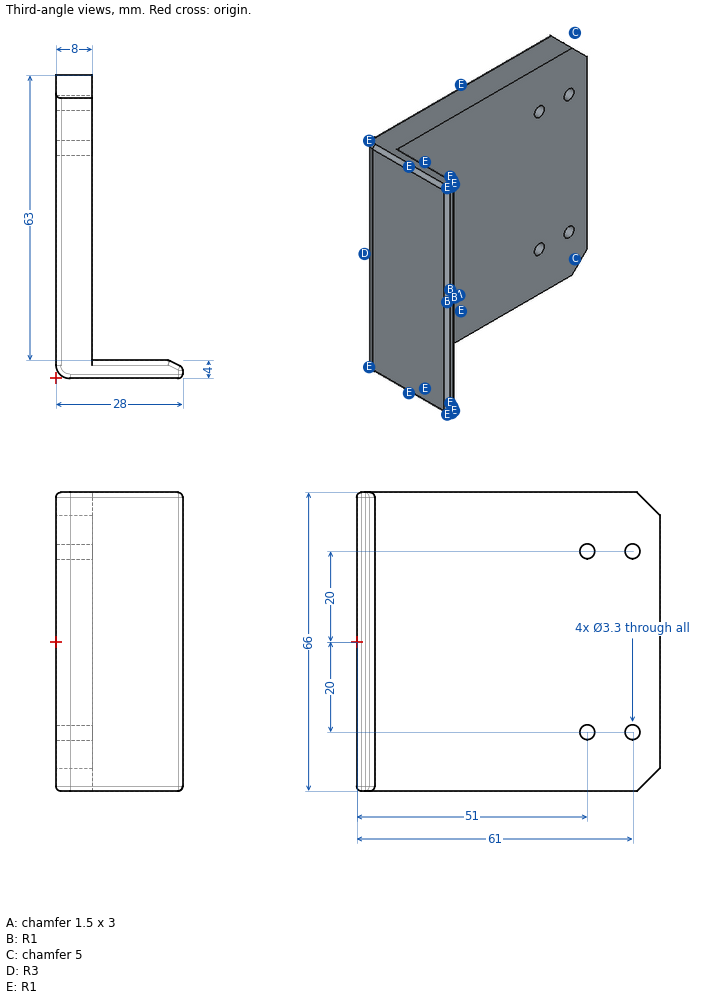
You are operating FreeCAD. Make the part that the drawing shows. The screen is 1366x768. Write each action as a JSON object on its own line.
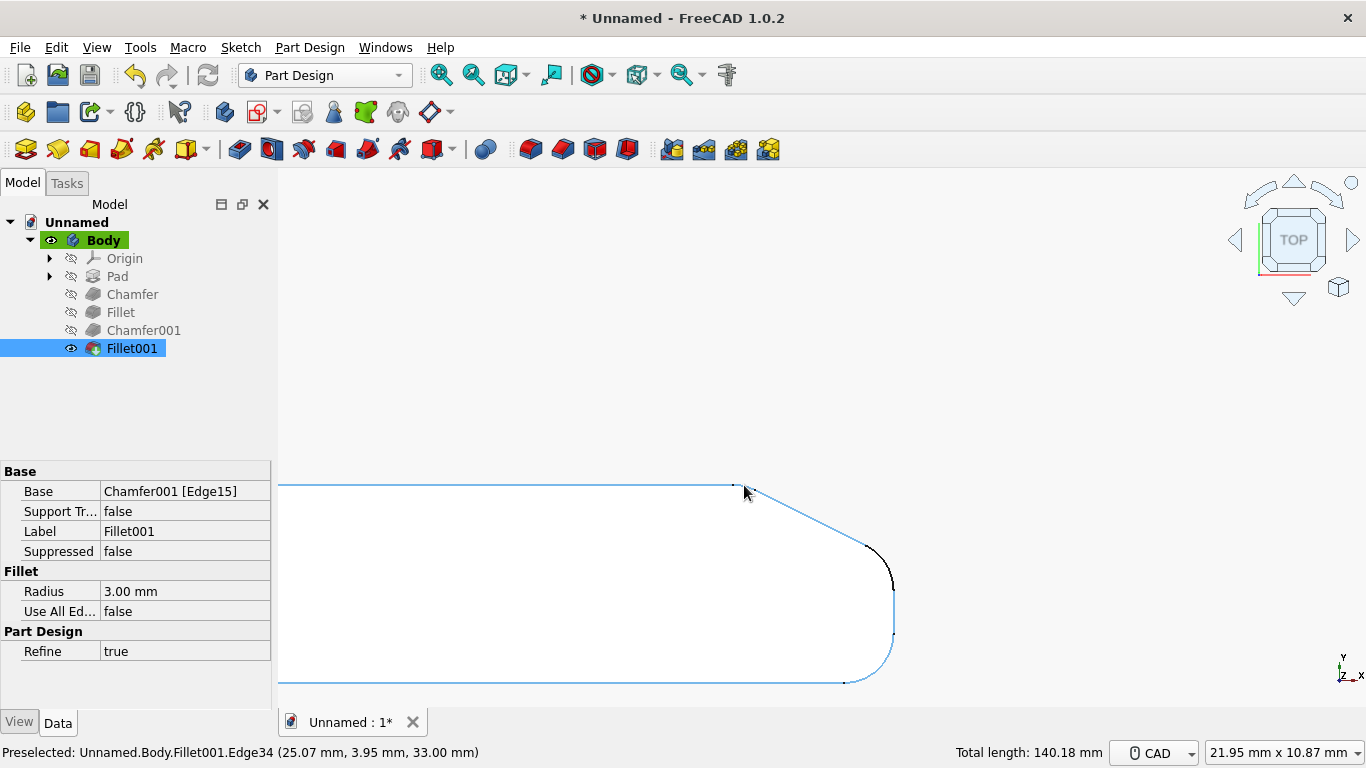
{"action": "left_click", "coordinate": [886, 563], "text": "ctrl"}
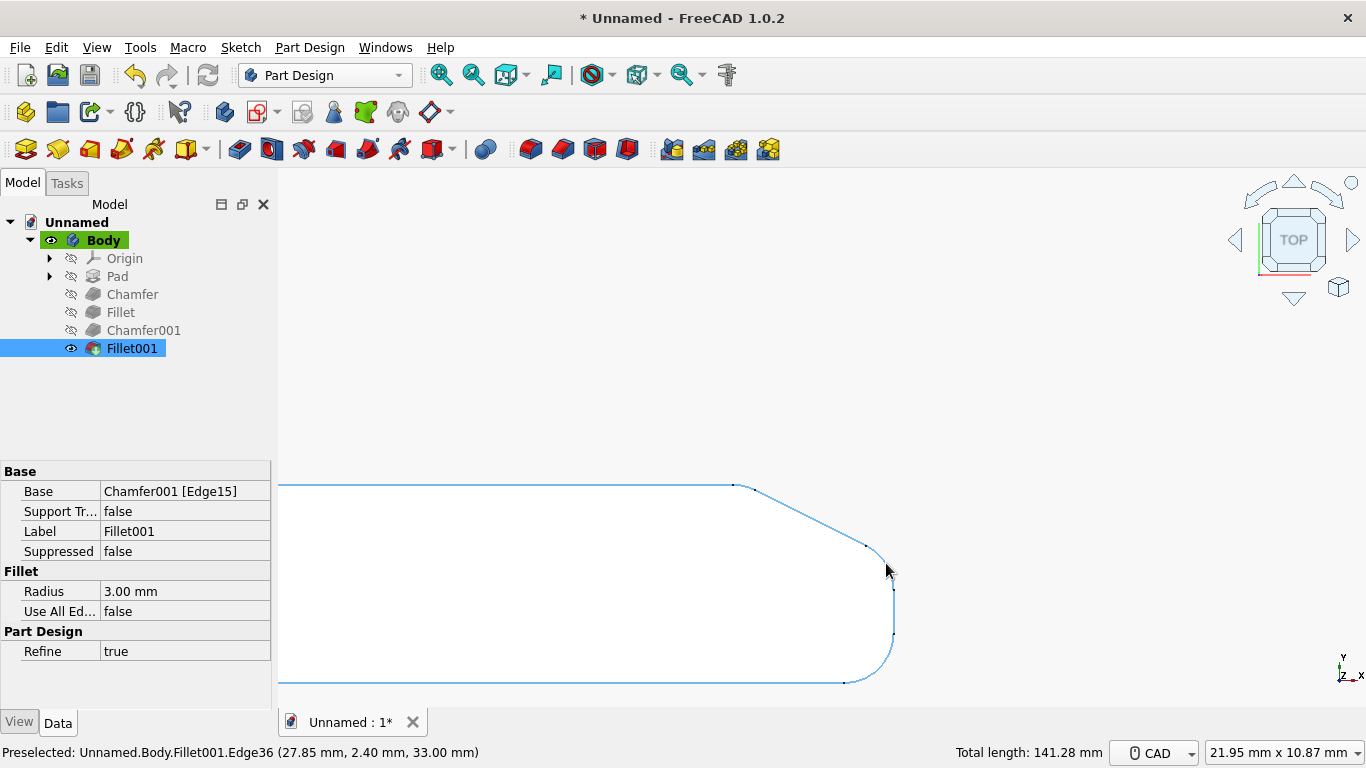
{"action": "left_click", "coordinate": [442, 76]}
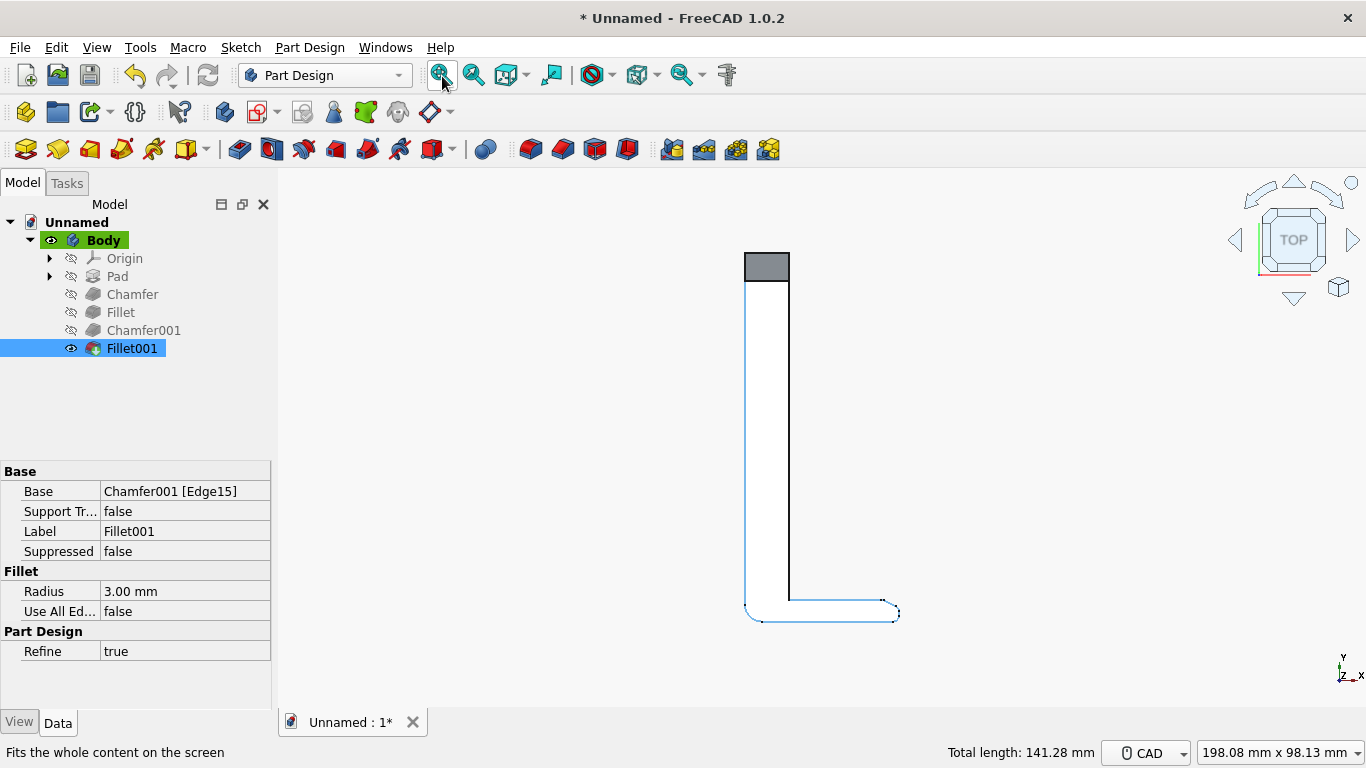
{"action": "key", "text": "1"}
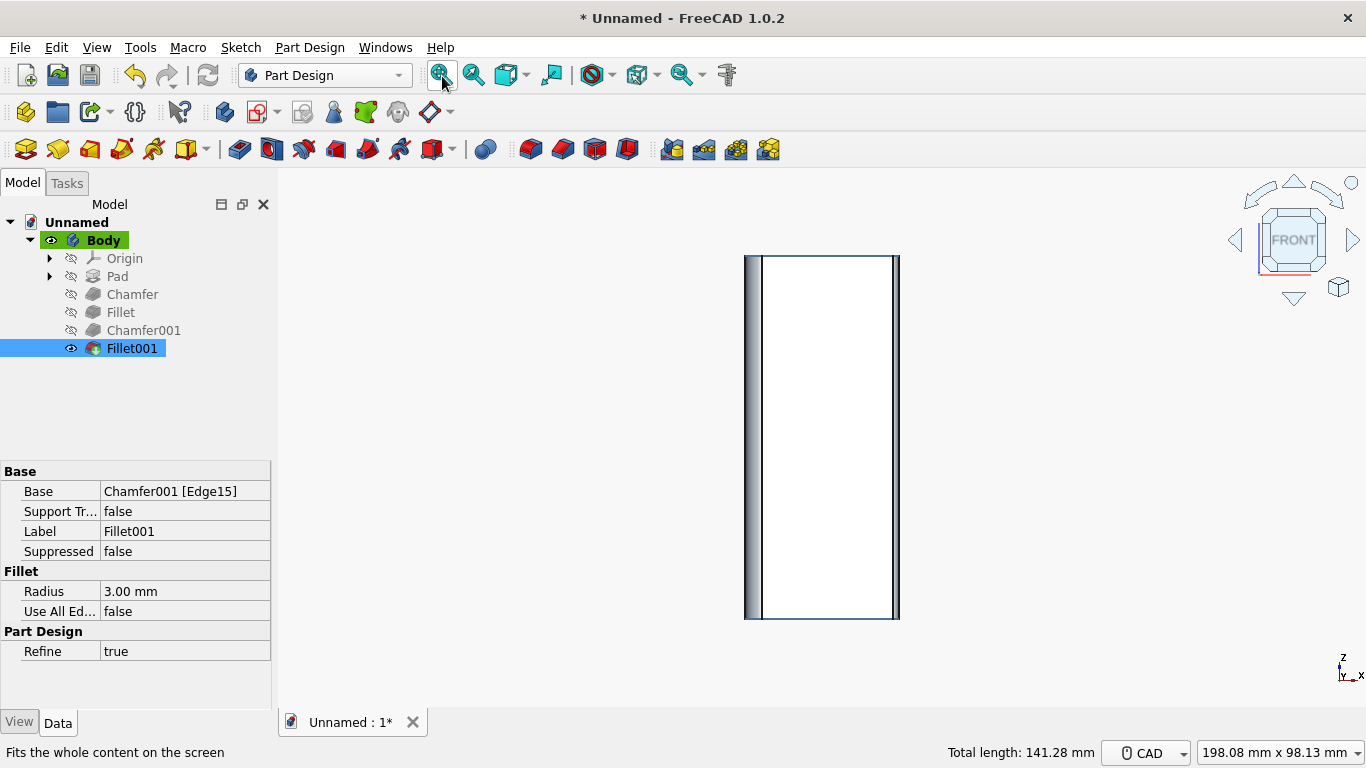
{"action": "scroll", "coordinate": [899, 618], "scroll_direction": "up", "scroll_amount": 11}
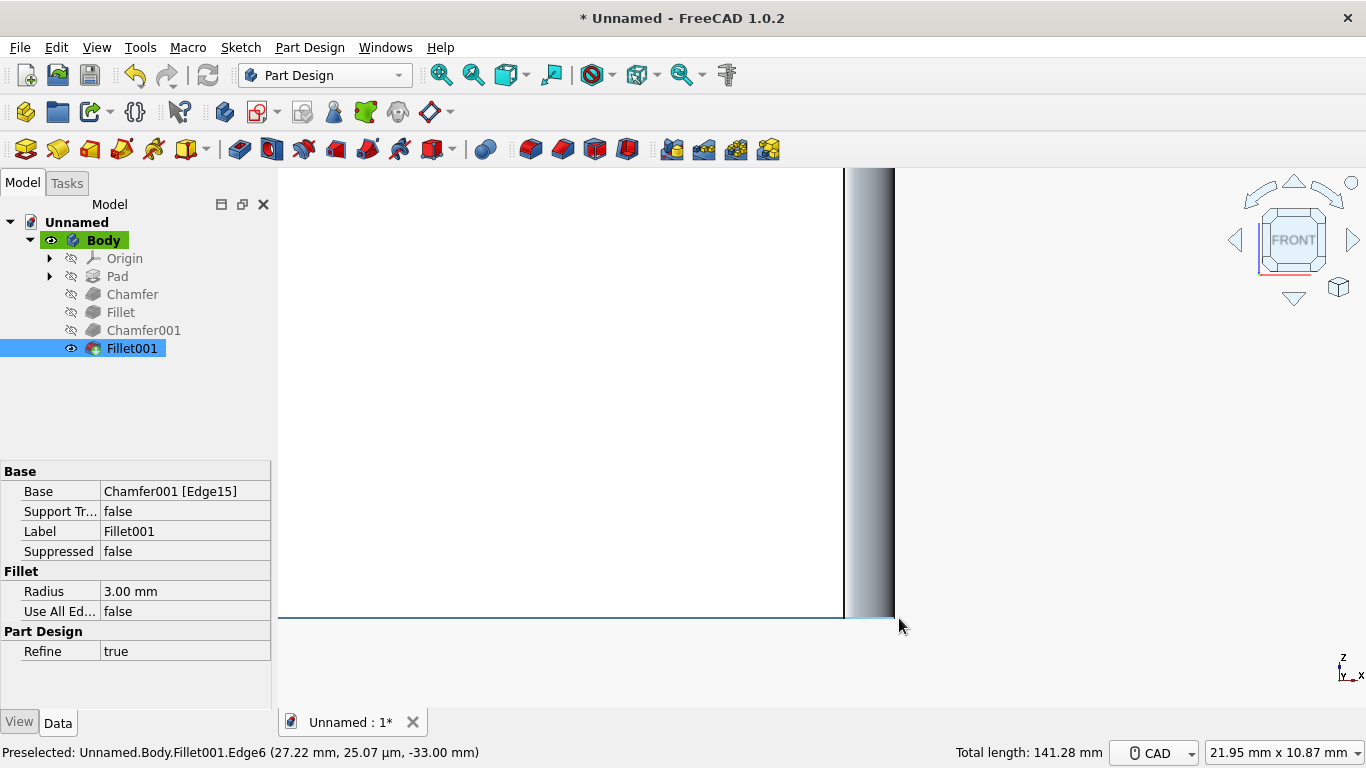
{"action": "key", "text": "v f"}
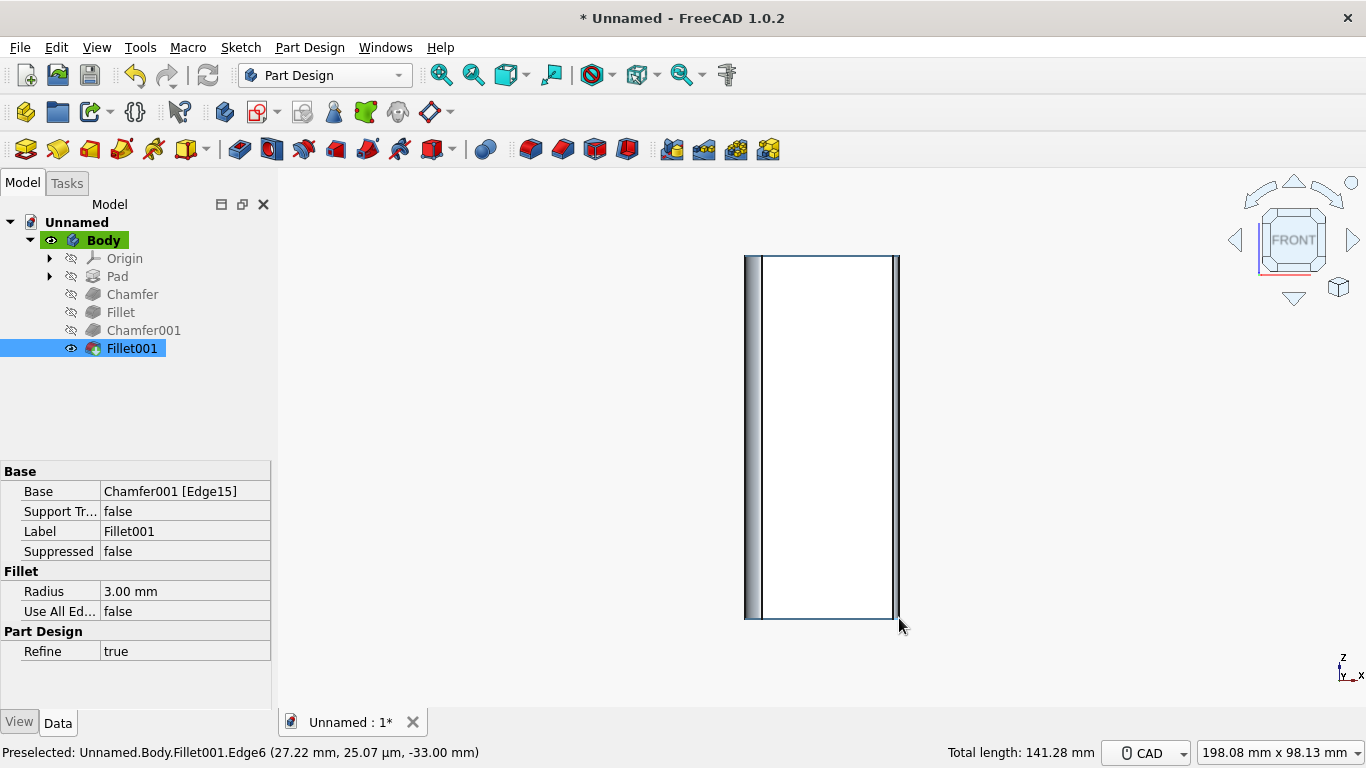
{"action": "key", "text": "3"}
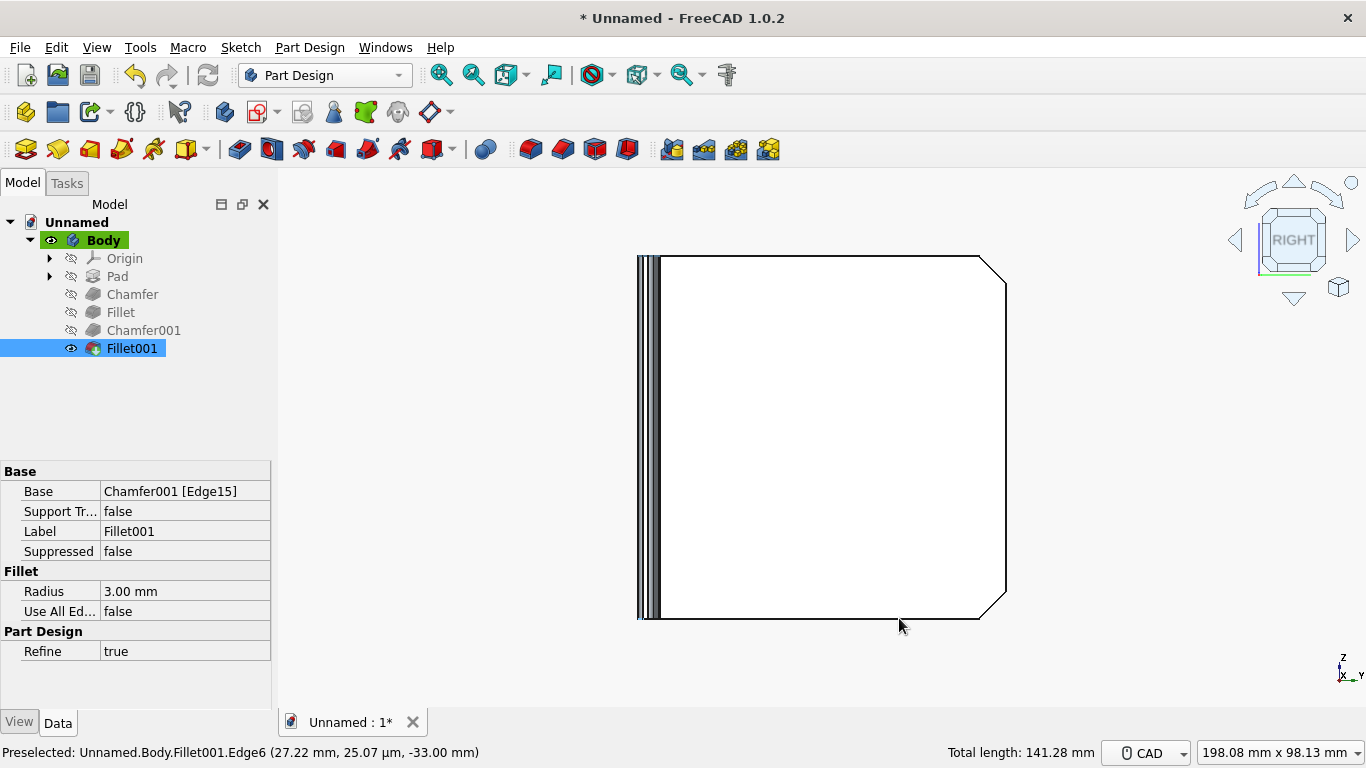
{"action": "scroll", "coordinate": [646, 618], "scroll_direction": "up", "scroll_amount": 11}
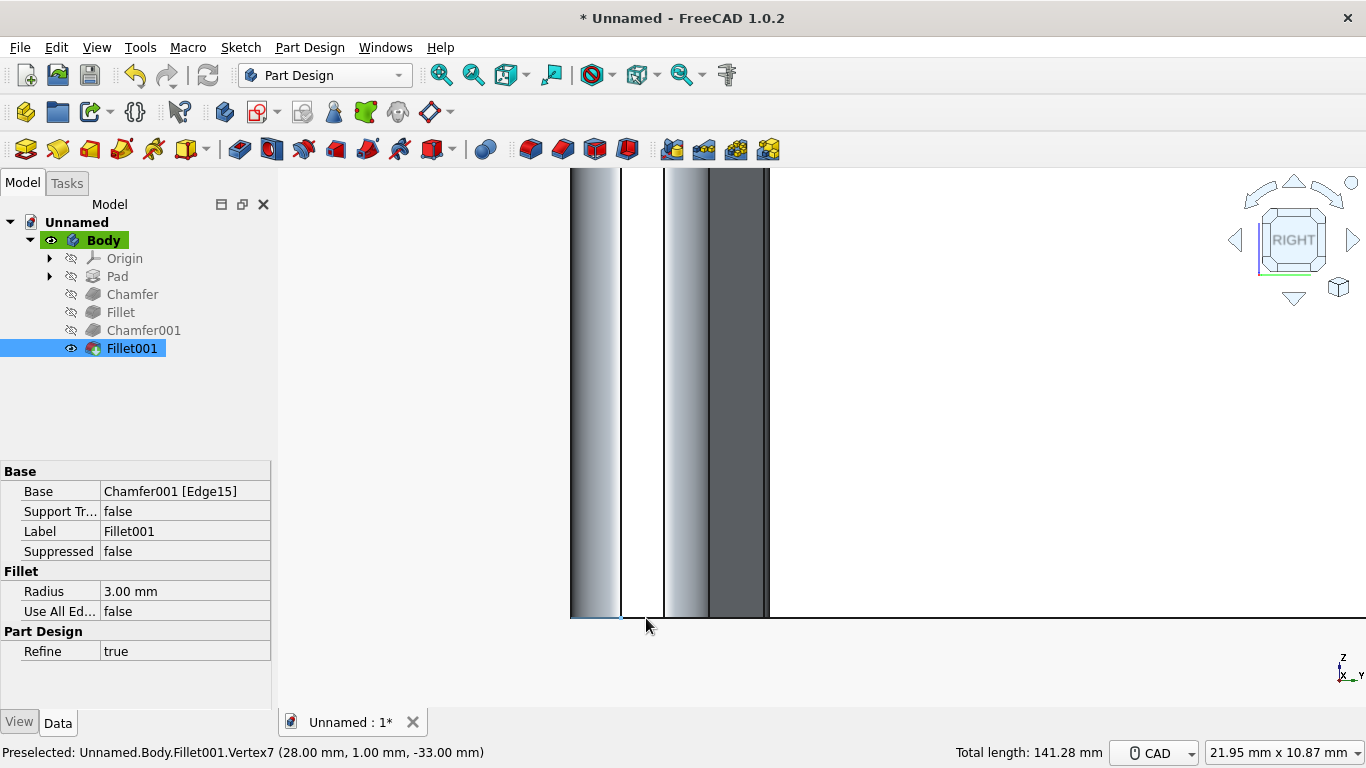
{"action": "left_click", "coordinate": [642, 617], "text": "ctrl"}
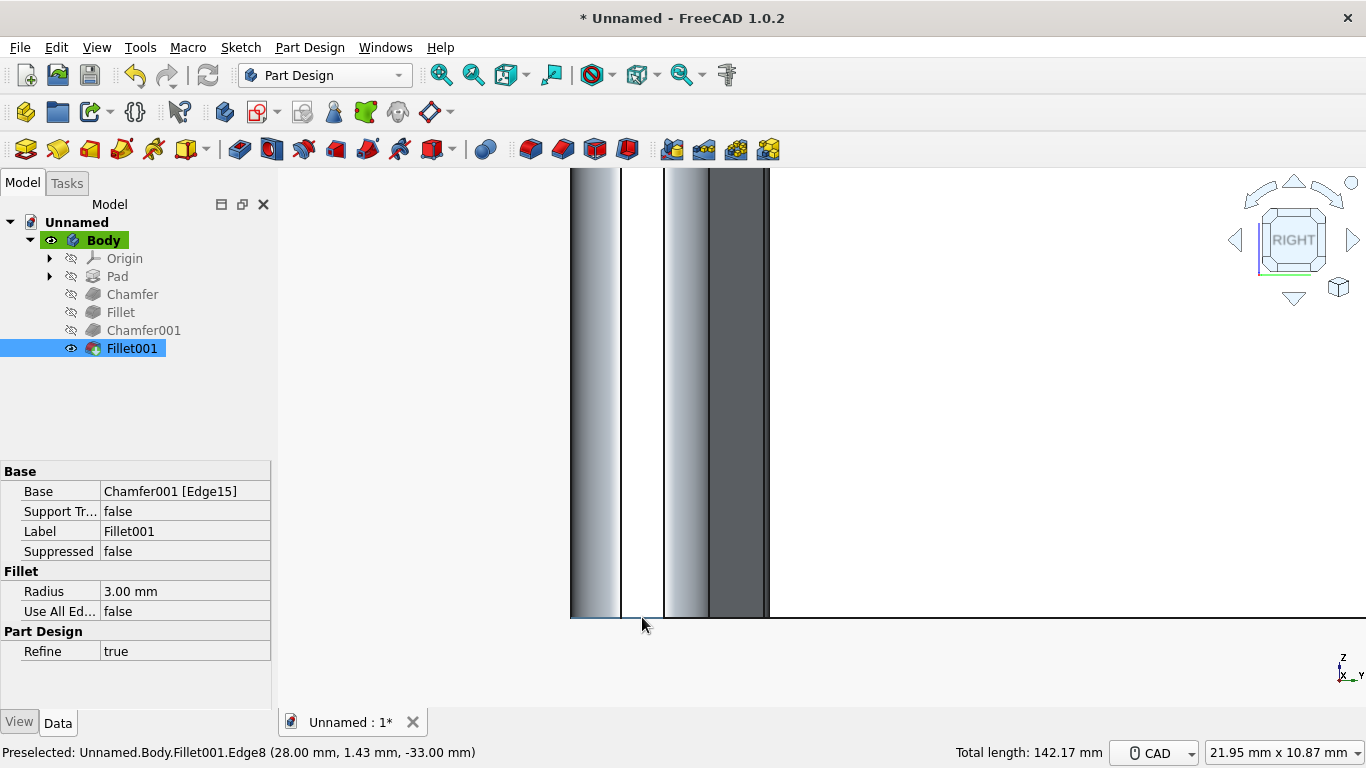
{"action": "left_click", "coordinate": [736, 617], "text": "ctrl"}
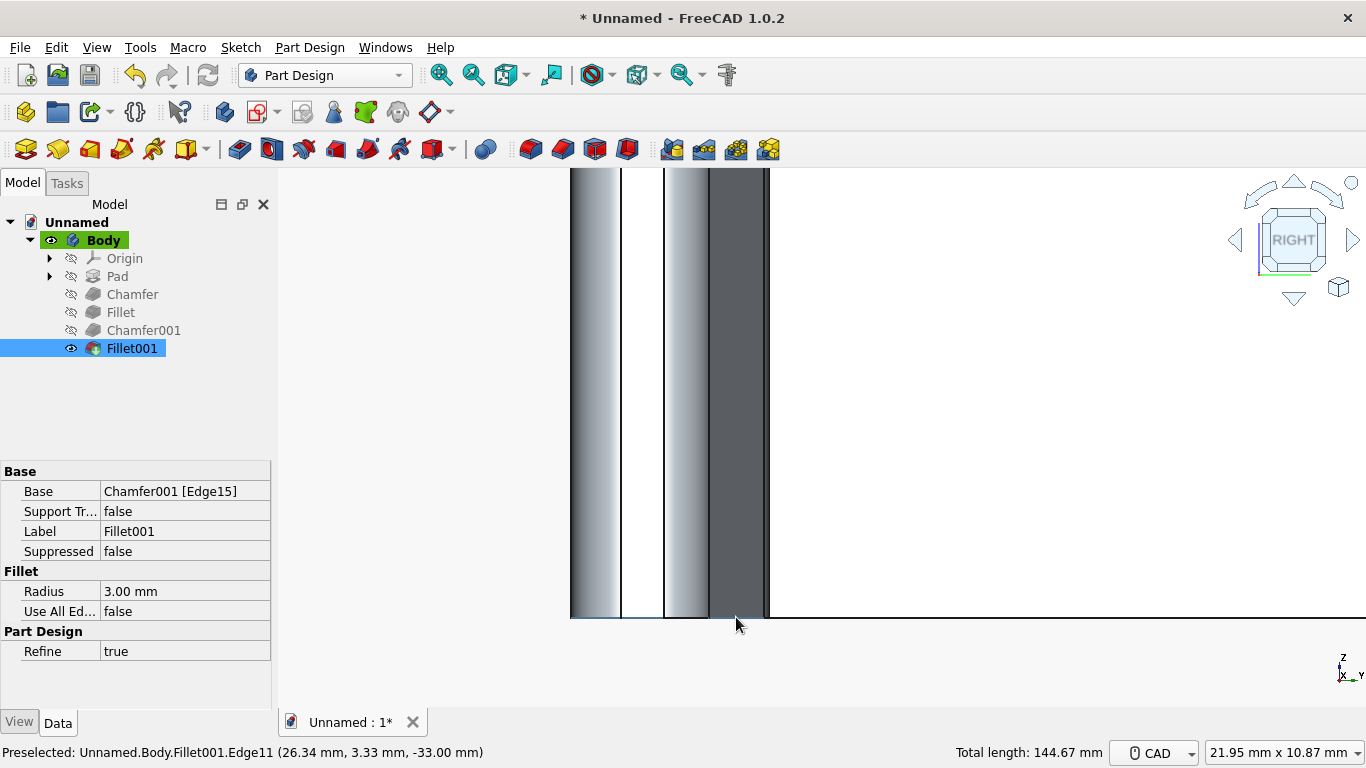
{"action": "left_click", "coordinate": [690, 617], "text": "ctrl"}